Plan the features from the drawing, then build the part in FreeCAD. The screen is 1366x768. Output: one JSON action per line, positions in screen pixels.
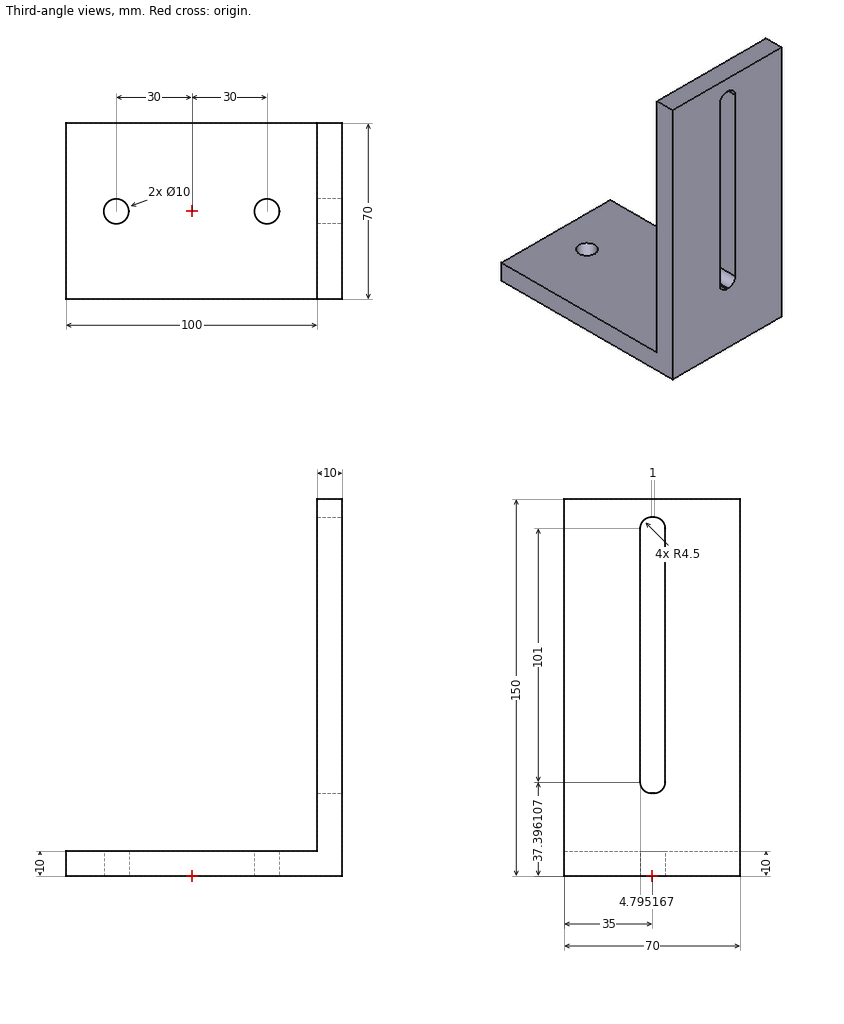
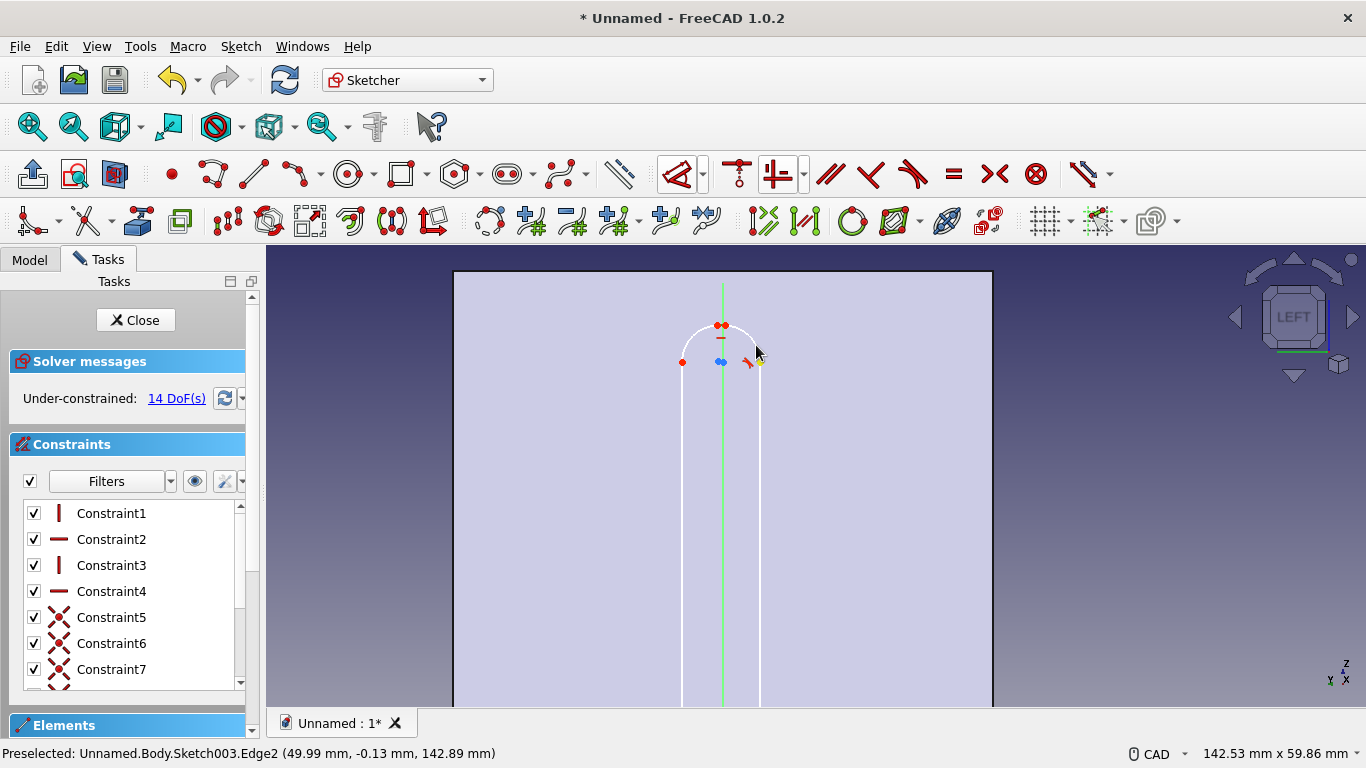
{"action": "left_click", "coordinate": [756, 346]}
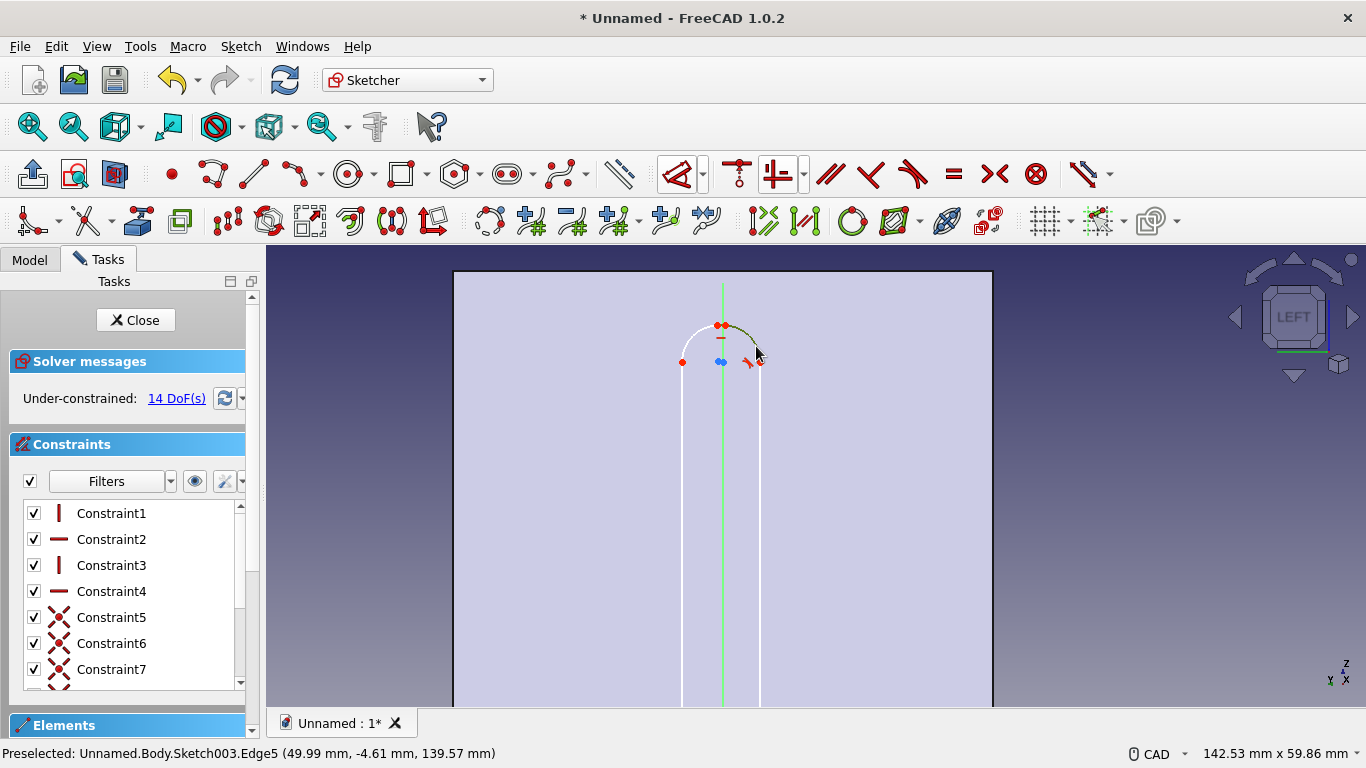
{"action": "left_click", "coordinate": [913, 174]}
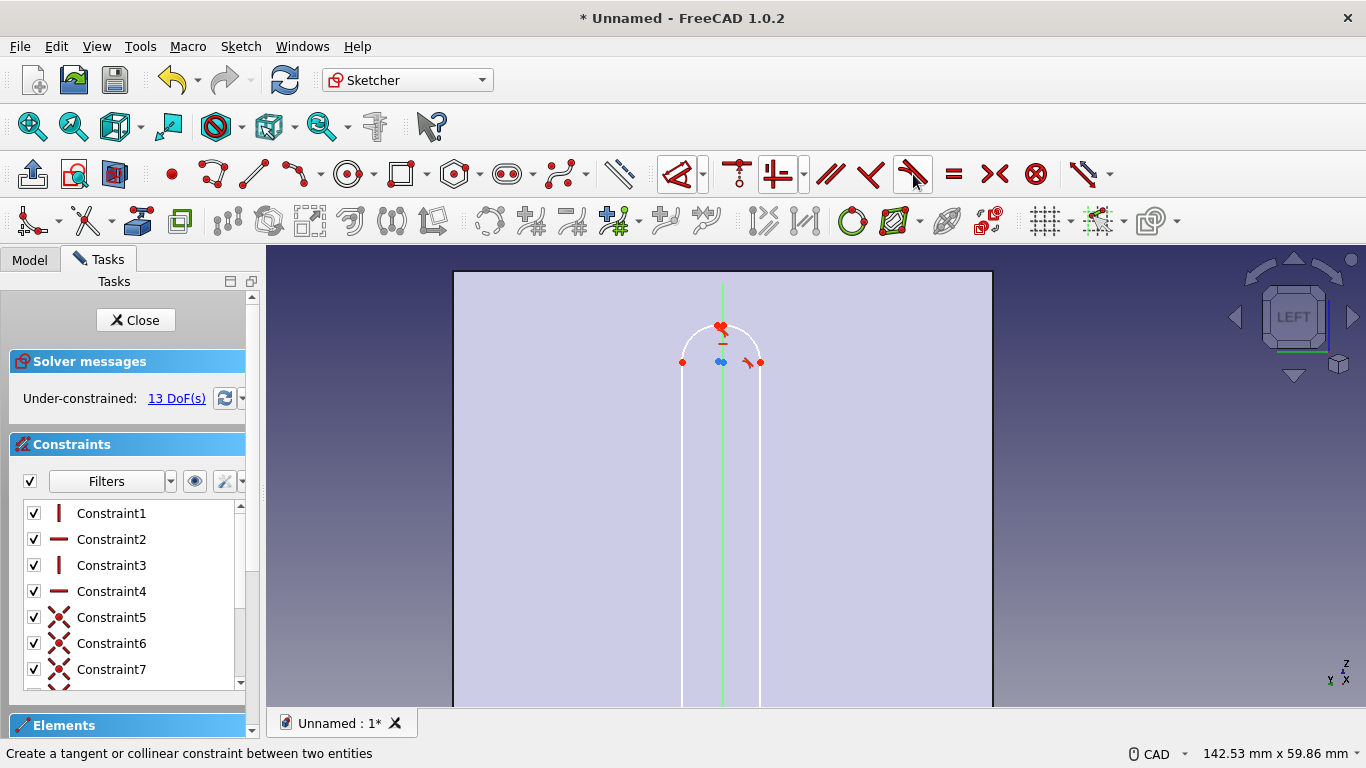
{"action": "scroll", "coordinate": [720, 325], "scroll_direction": "up", "scroll_amount": 8}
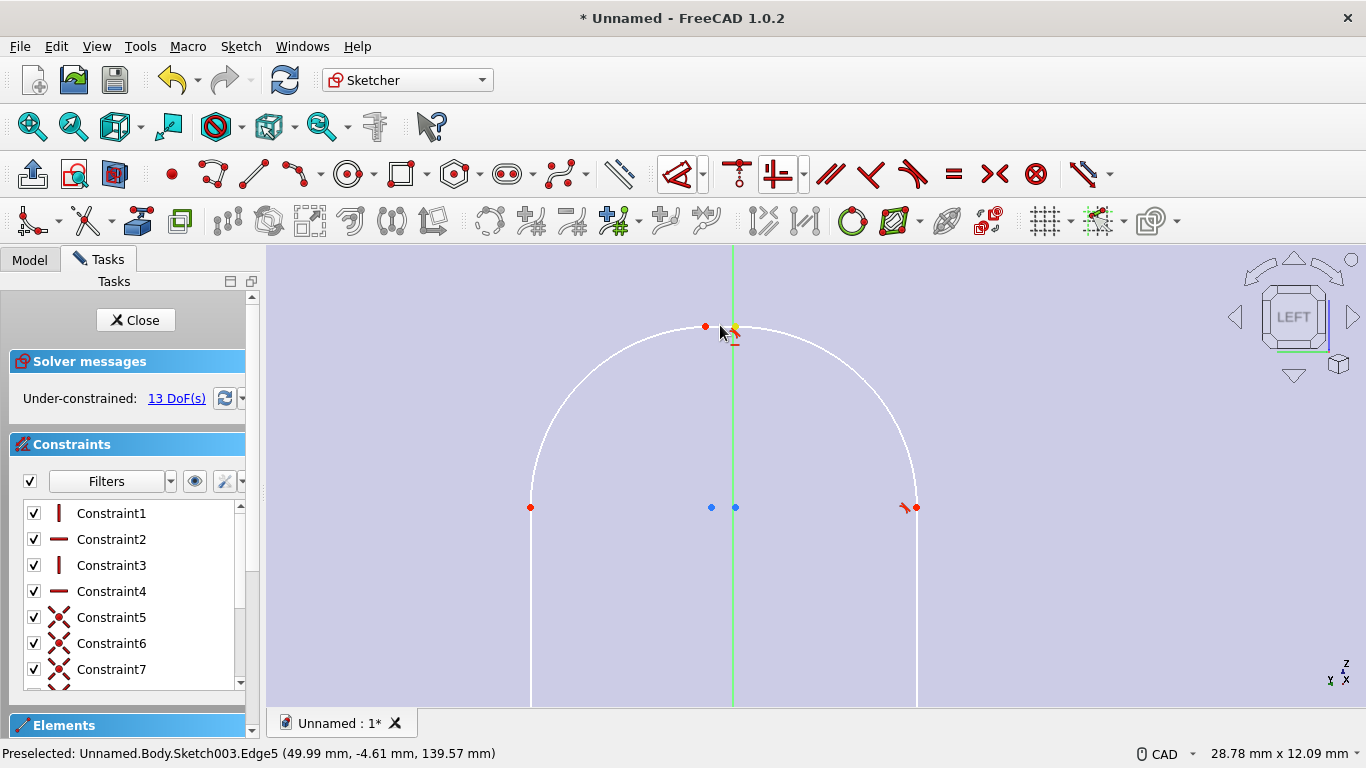
{"action": "left_click", "coordinate": [721, 327]}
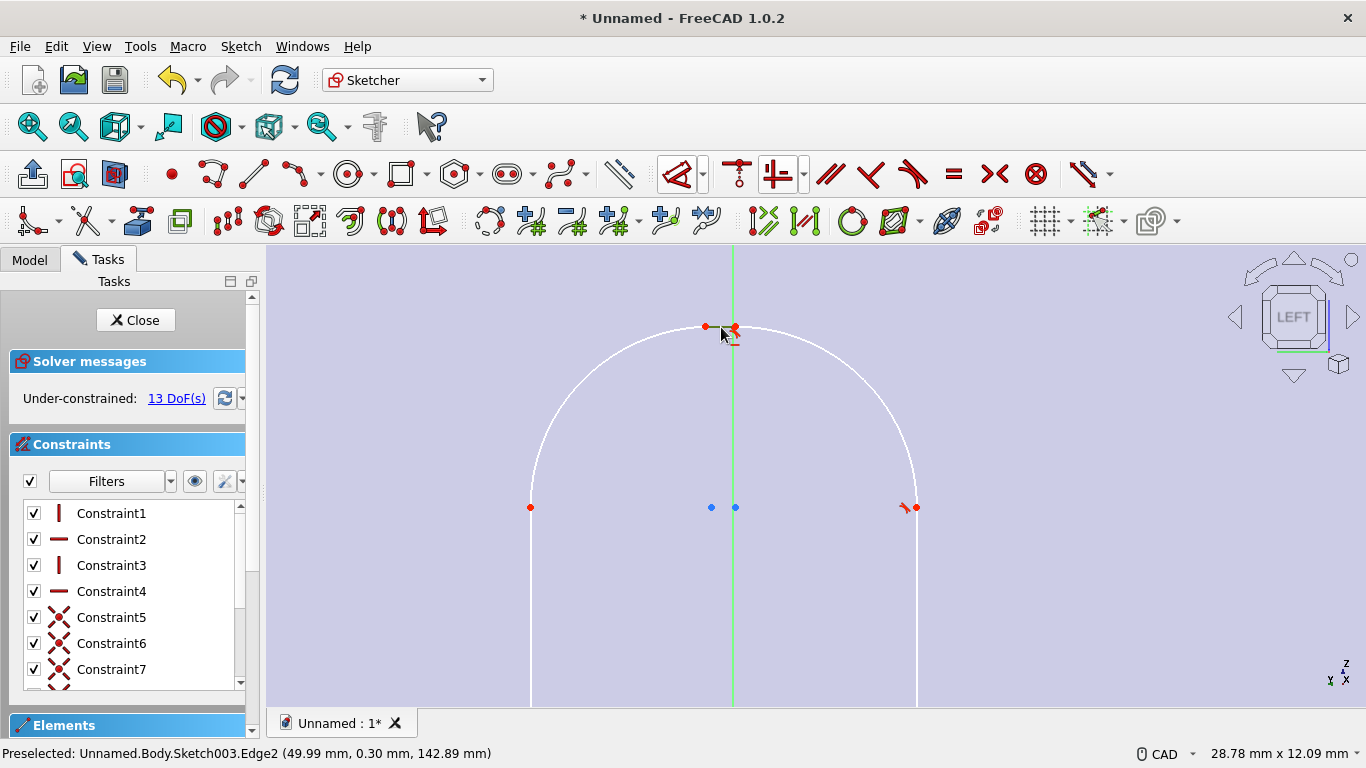
{"action": "scroll", "coordinate": [749, 341], "scroll_direction": "down", "scroll_amount": 15}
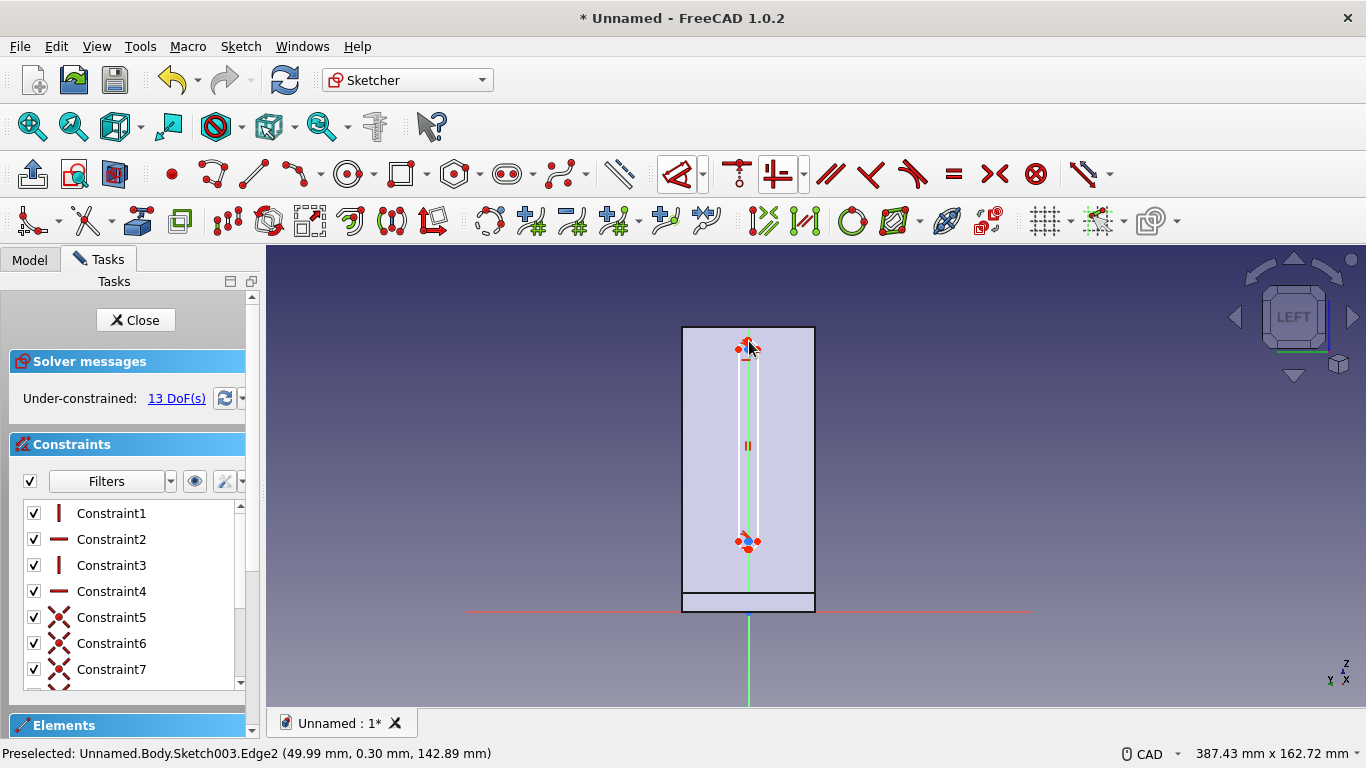
{"action": "scroll", "coordinate": [743, 342], "scroll_direction": "up", "scroll_amount": 7}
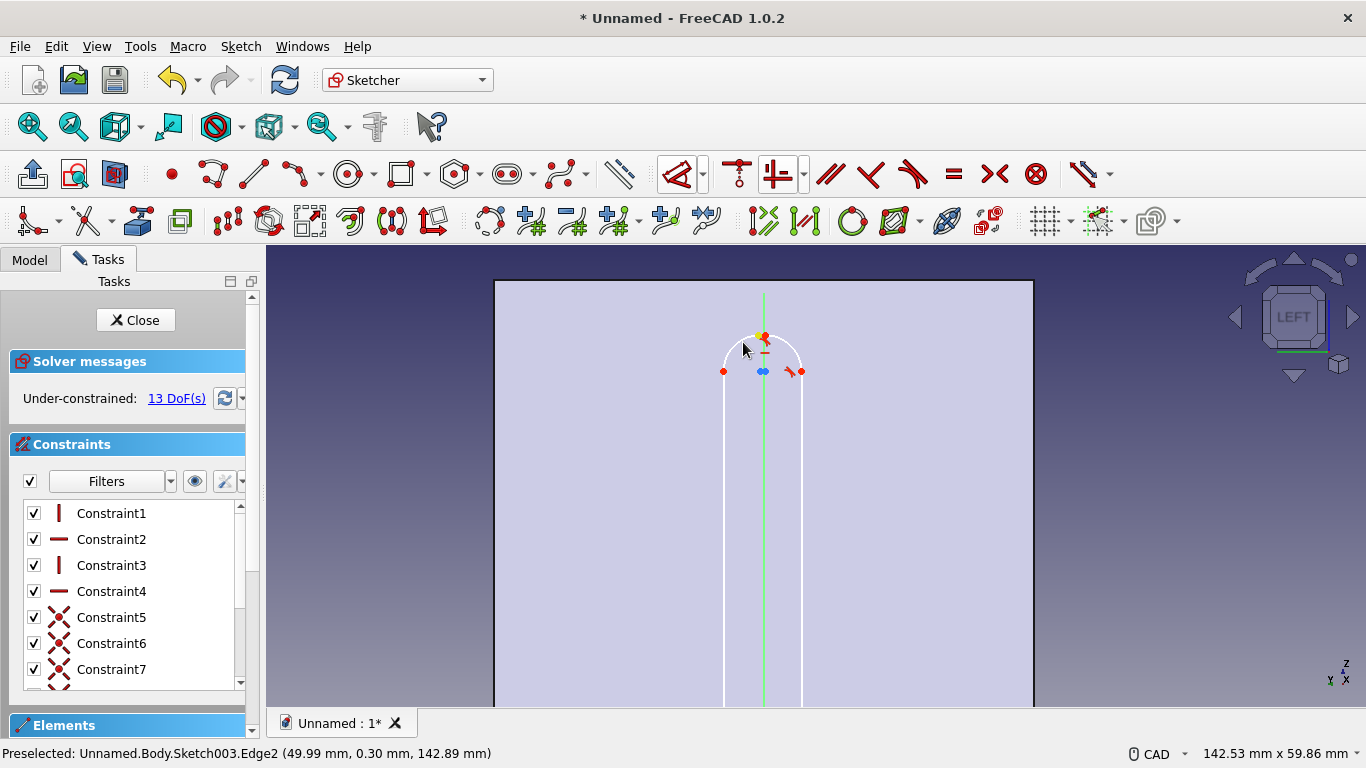
{"action": "left_click", "coordinate": [743, 340]}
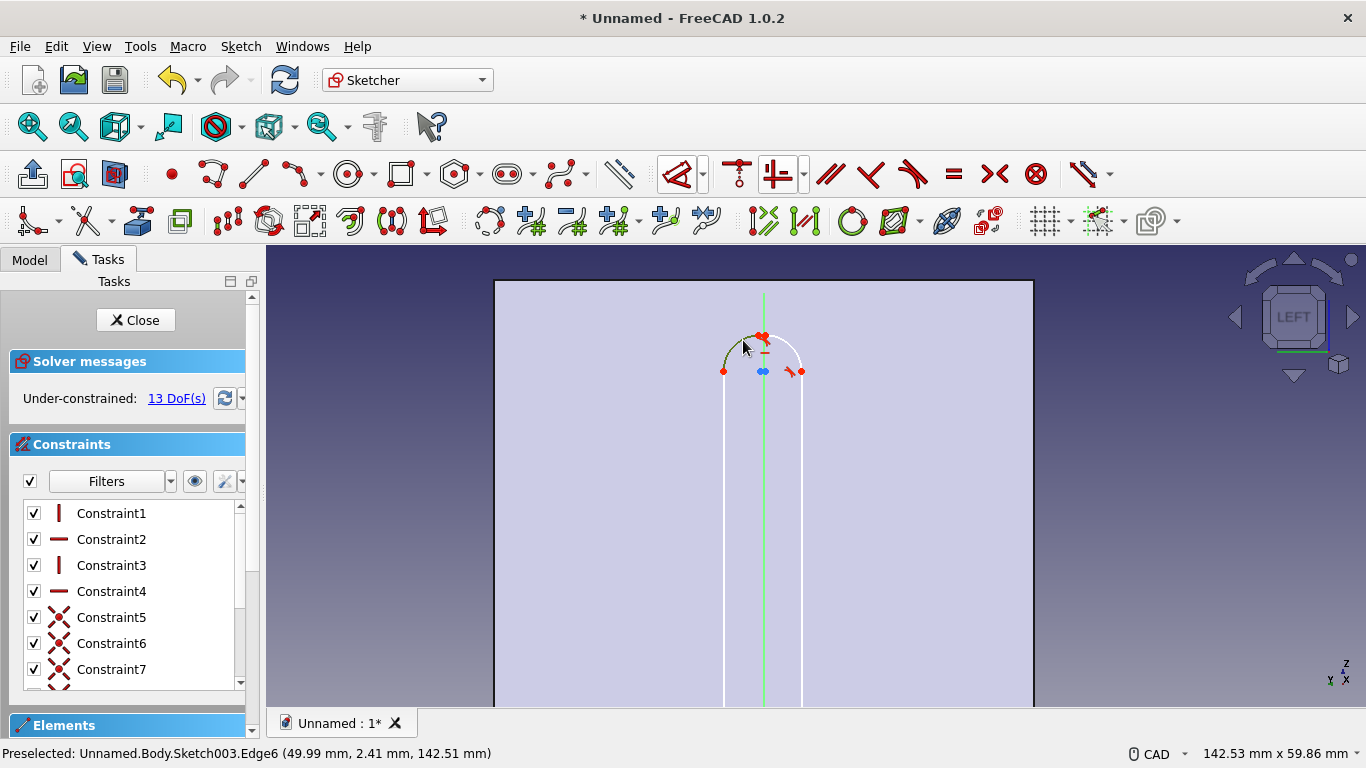
{"action": "left_click", "coordinate": [913, 174]}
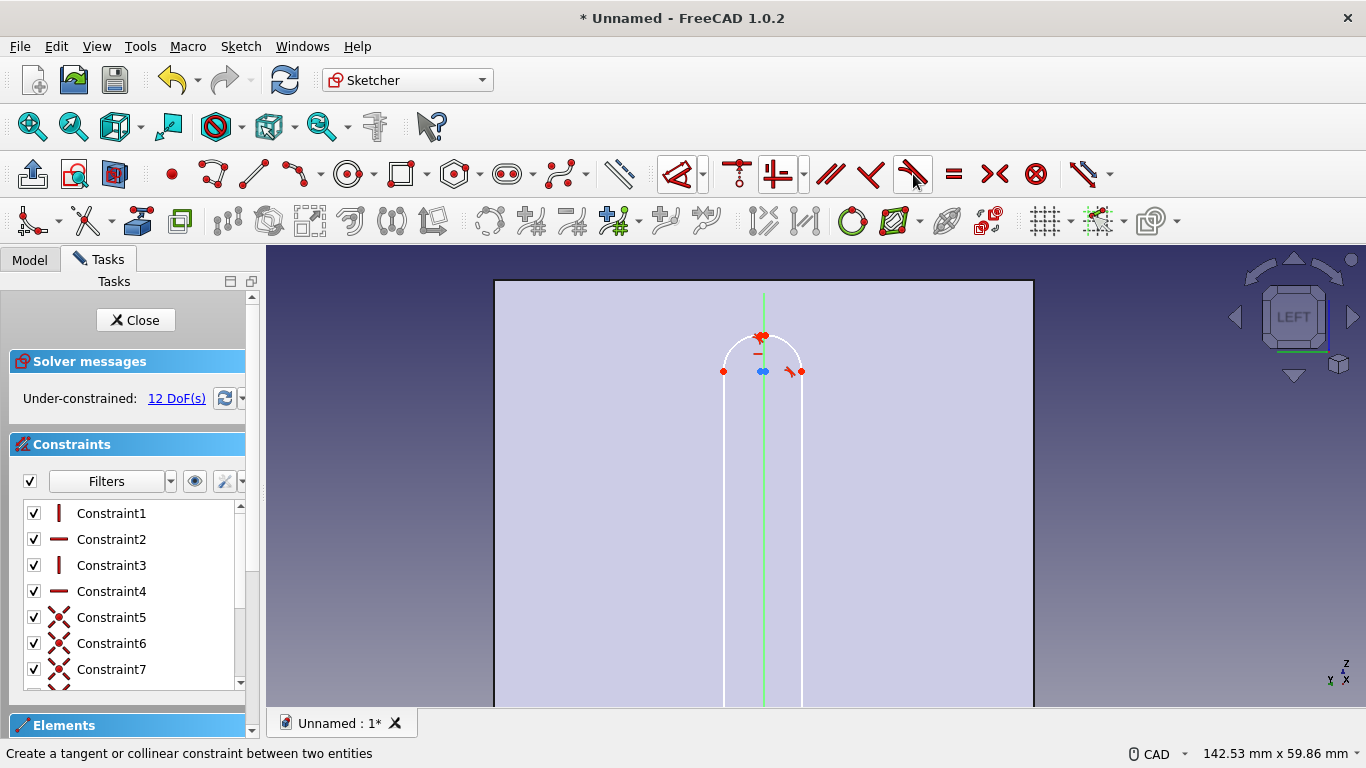
{"action": "left_click", "coordinate": [724, 606]}